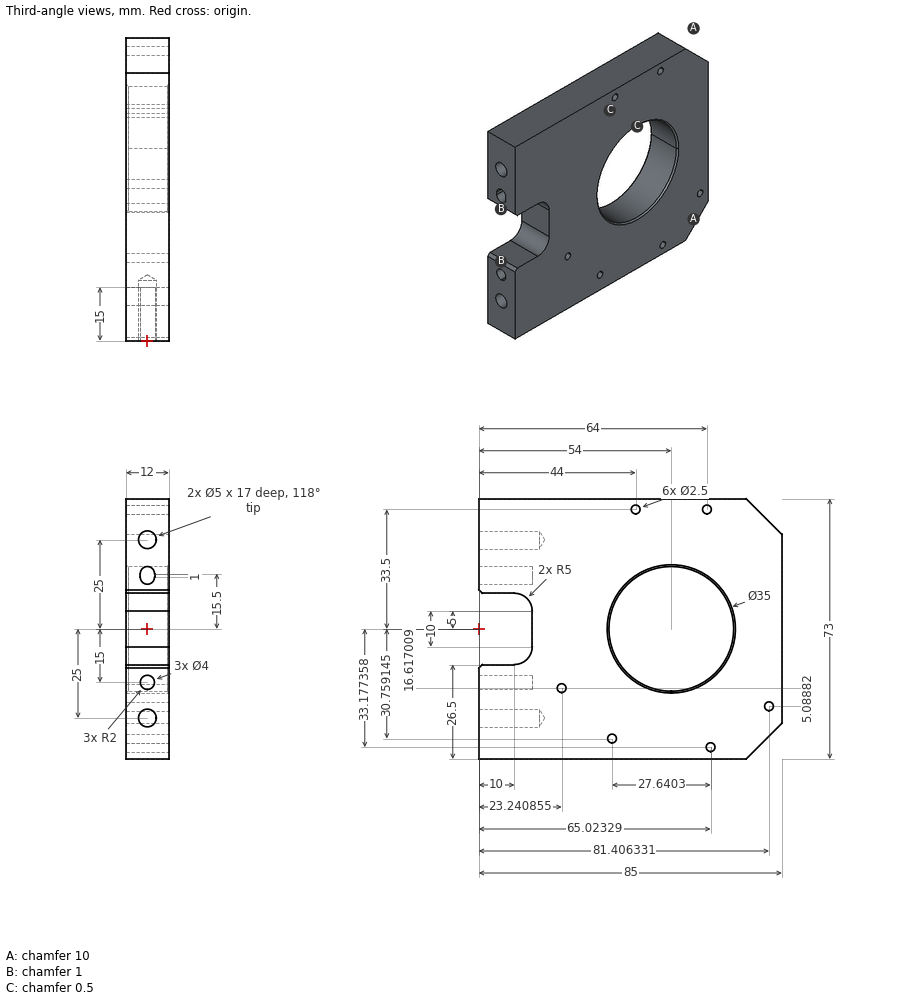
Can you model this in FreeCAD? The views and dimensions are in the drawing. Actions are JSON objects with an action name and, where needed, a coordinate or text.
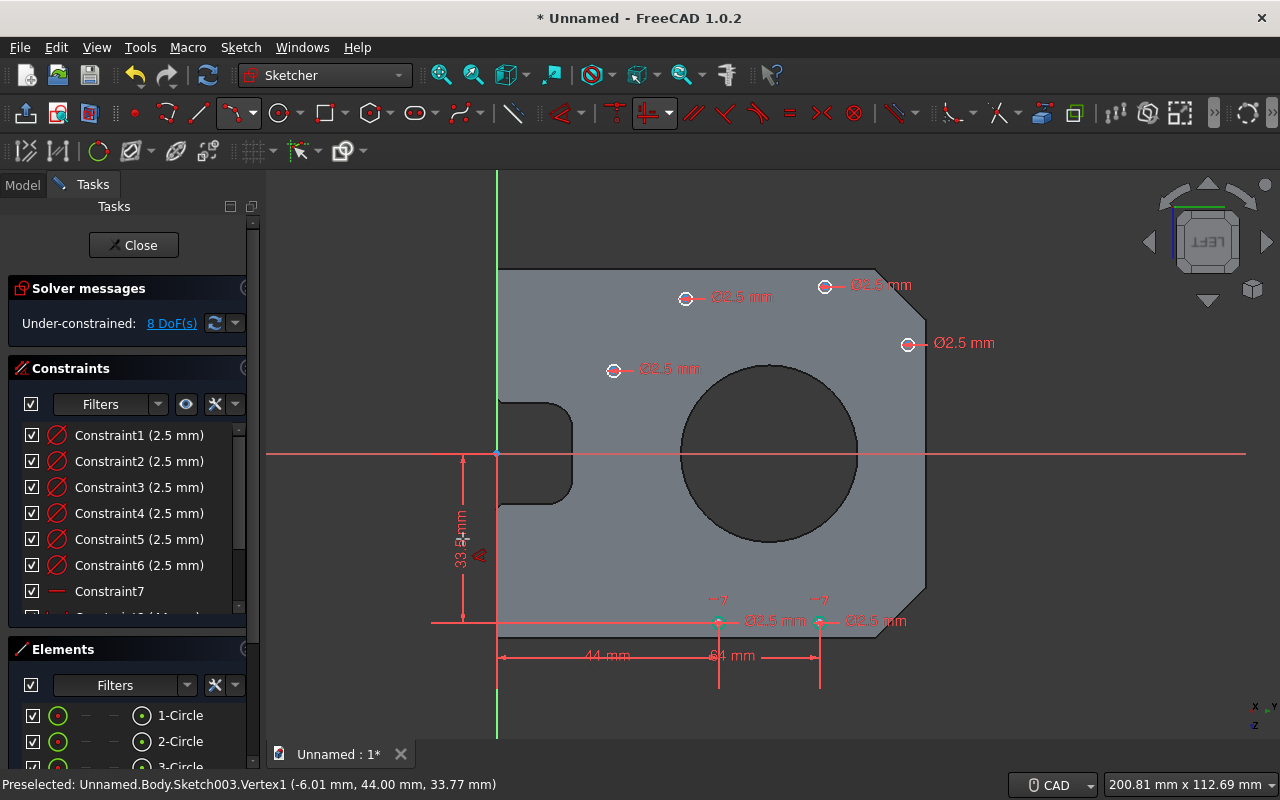
{"action": "left_click", "coordinate": [825, 287]}
{"action": "left_click", "coordinate": [661, 253]}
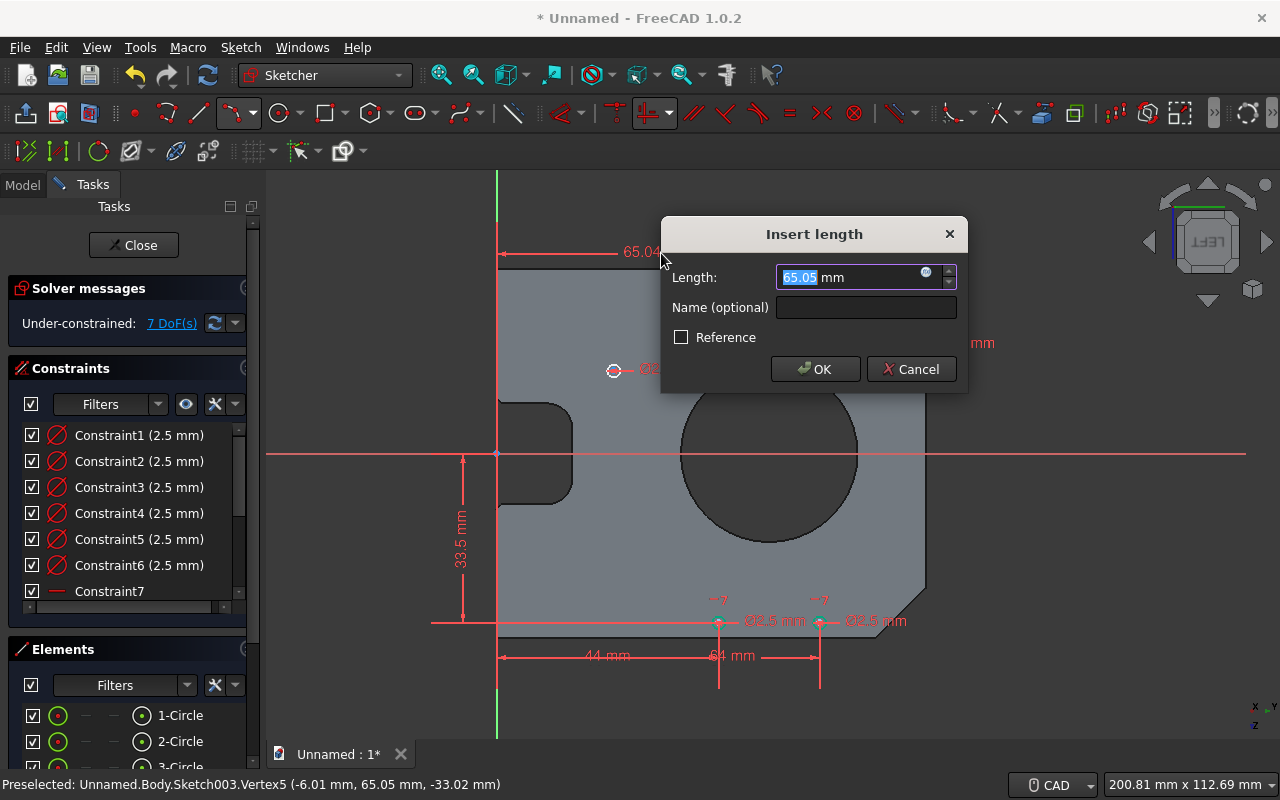
{"action": "type", "text": "65.02329"}
{"action": "key", "text": "Return"}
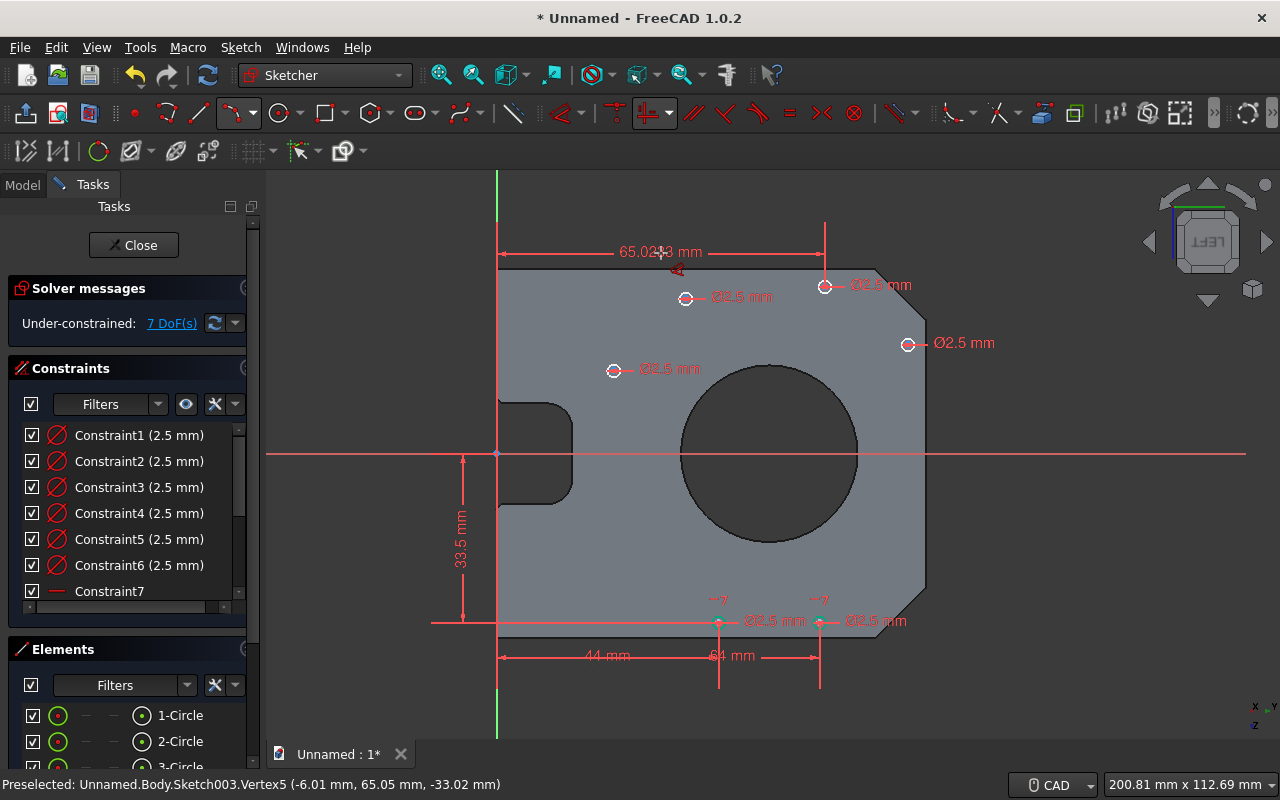
{"action": "left_click", "coordinate": [686, 299]}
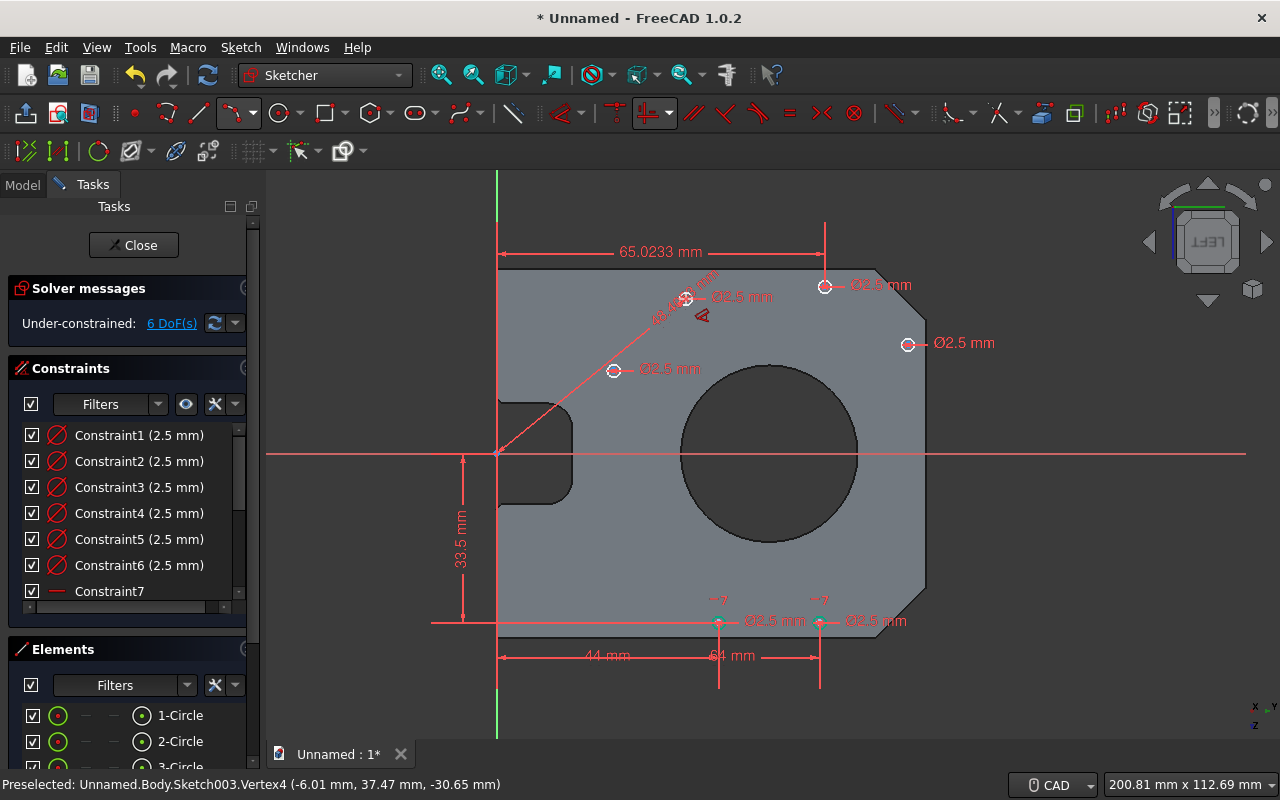
{"action": "left_click", "coordinate": [825, 287]}
{"action": "left_click", "coordinate": [755, 253]}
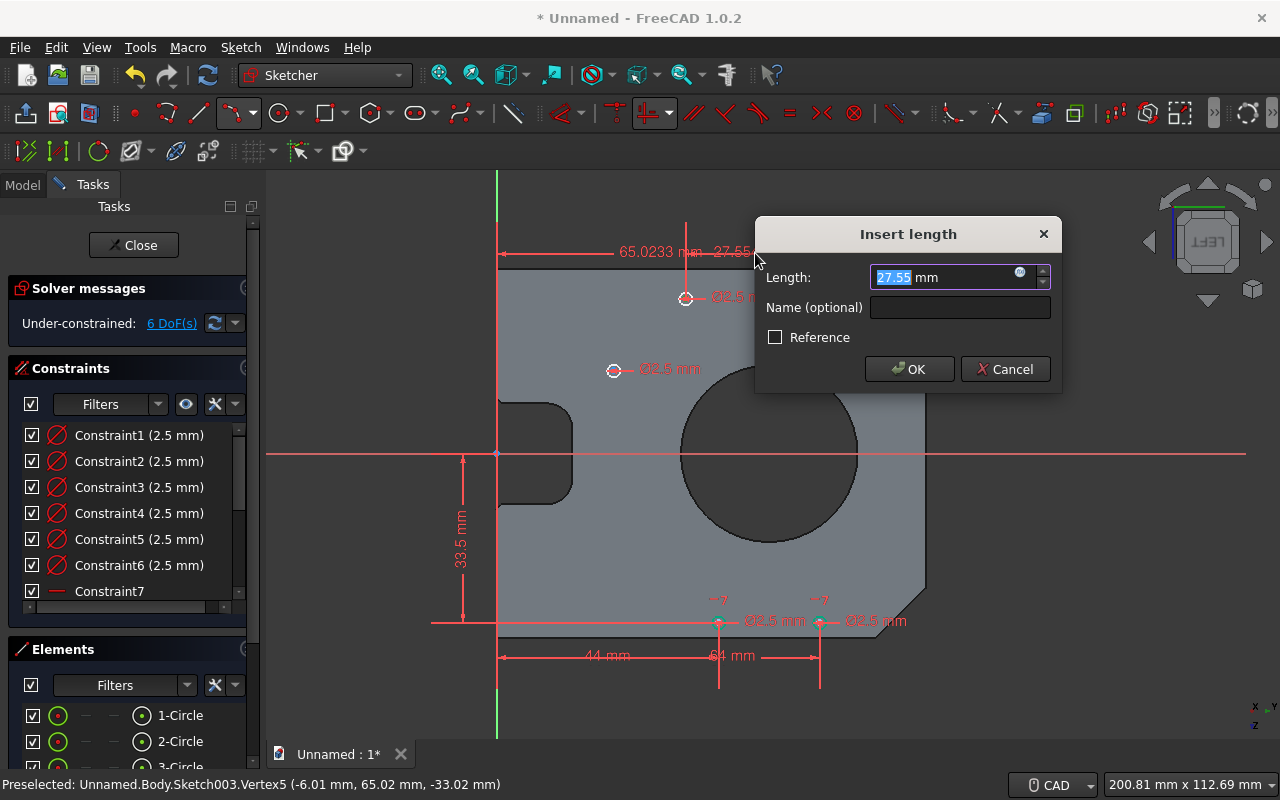
{"action": "type", "text": "27.6403"}
{"action": "key", "text": "Return"}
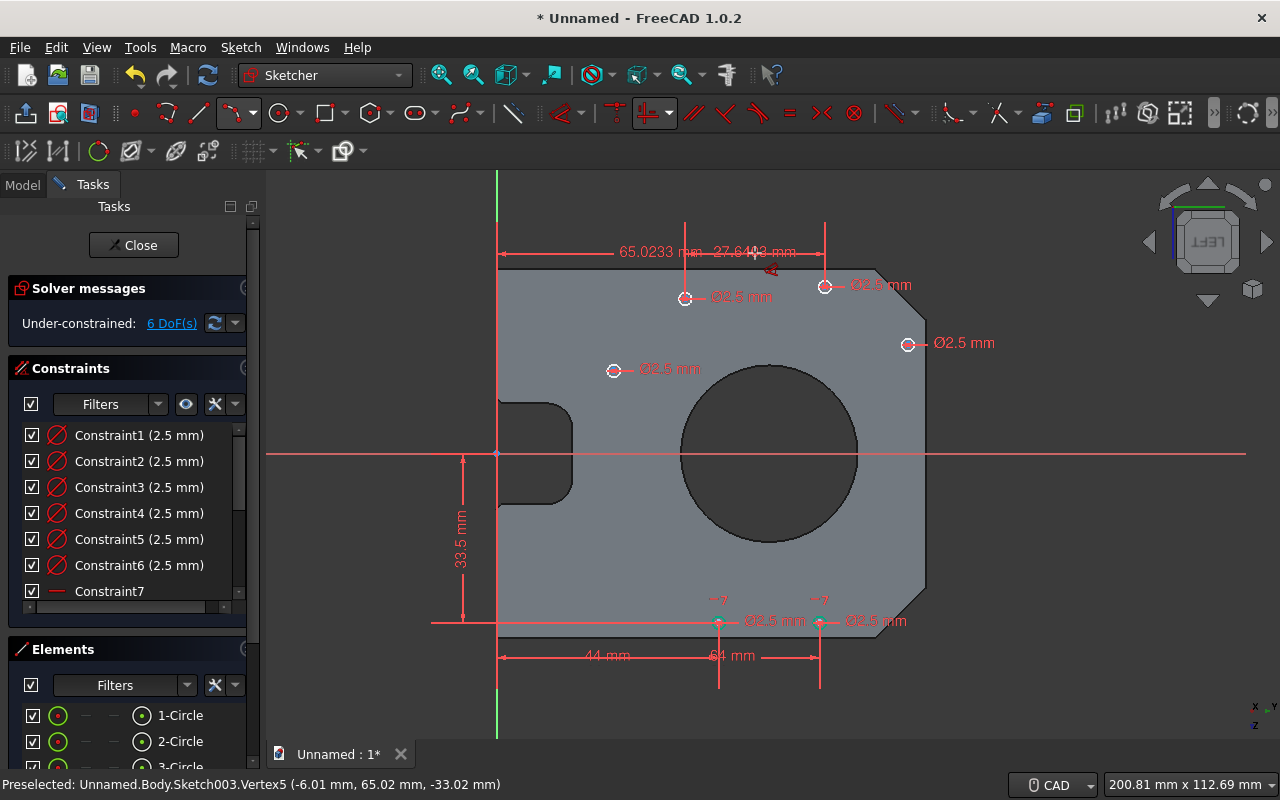
{"action": "scroll", "coordinate": [614, 371], "scroll_direction": "up", "scroll_amount": 3}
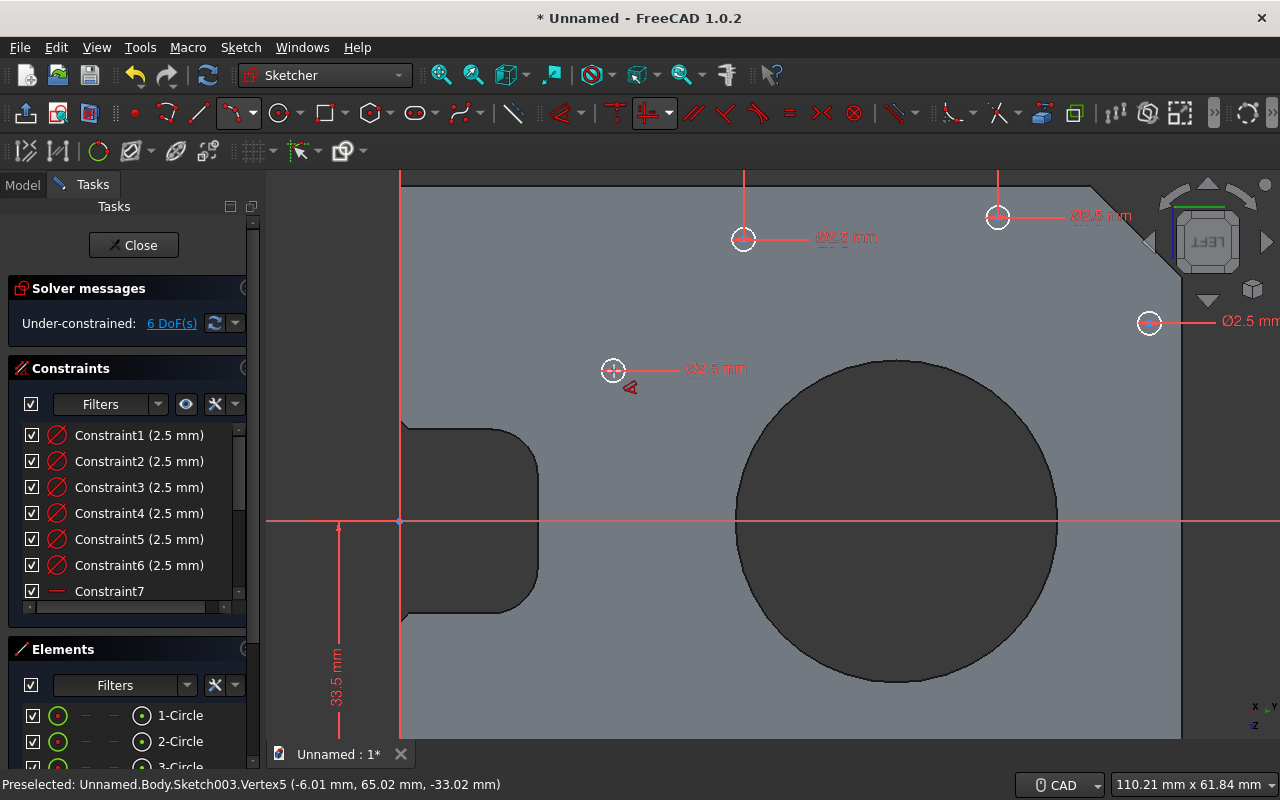
{"action": "left_click", "coordinate": [613, 371]}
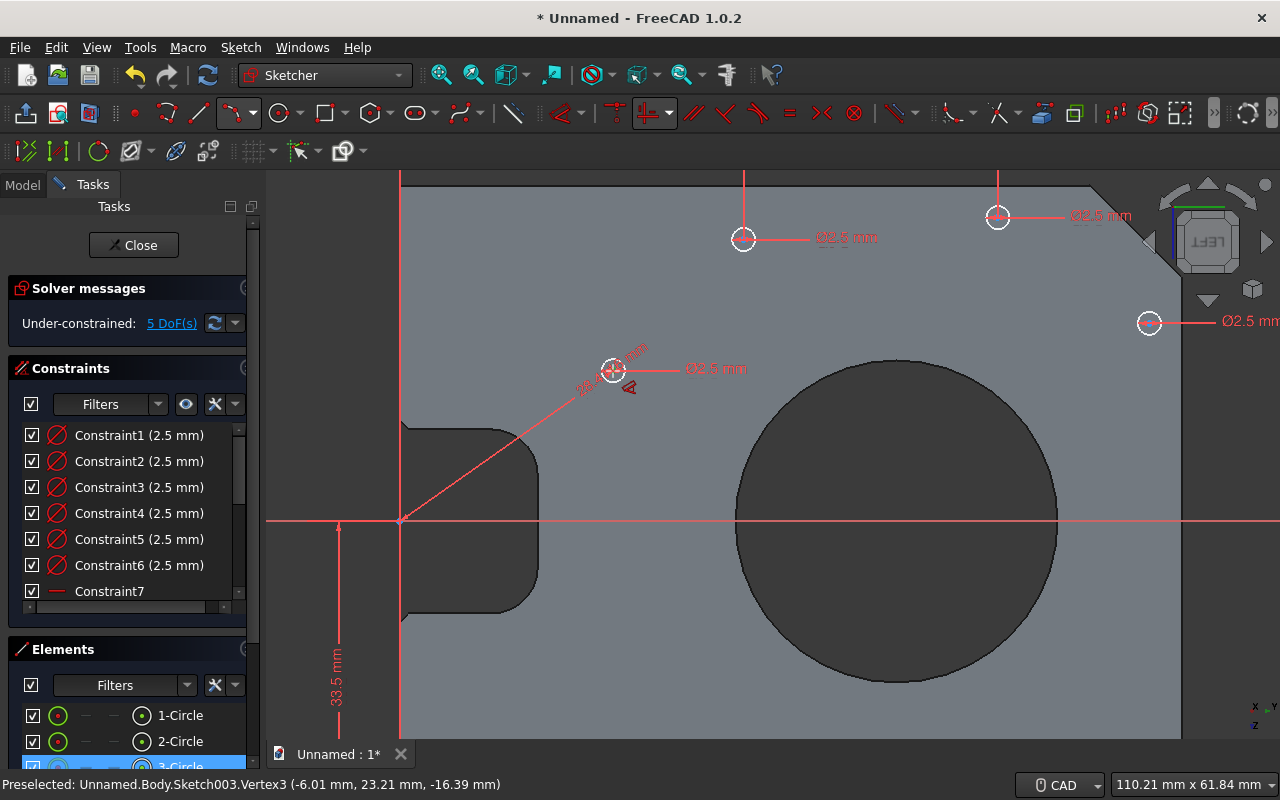
{"action": "scroll", "coordinate": [613, 371], "scroll_direction": "down", "scroll_amount": 3}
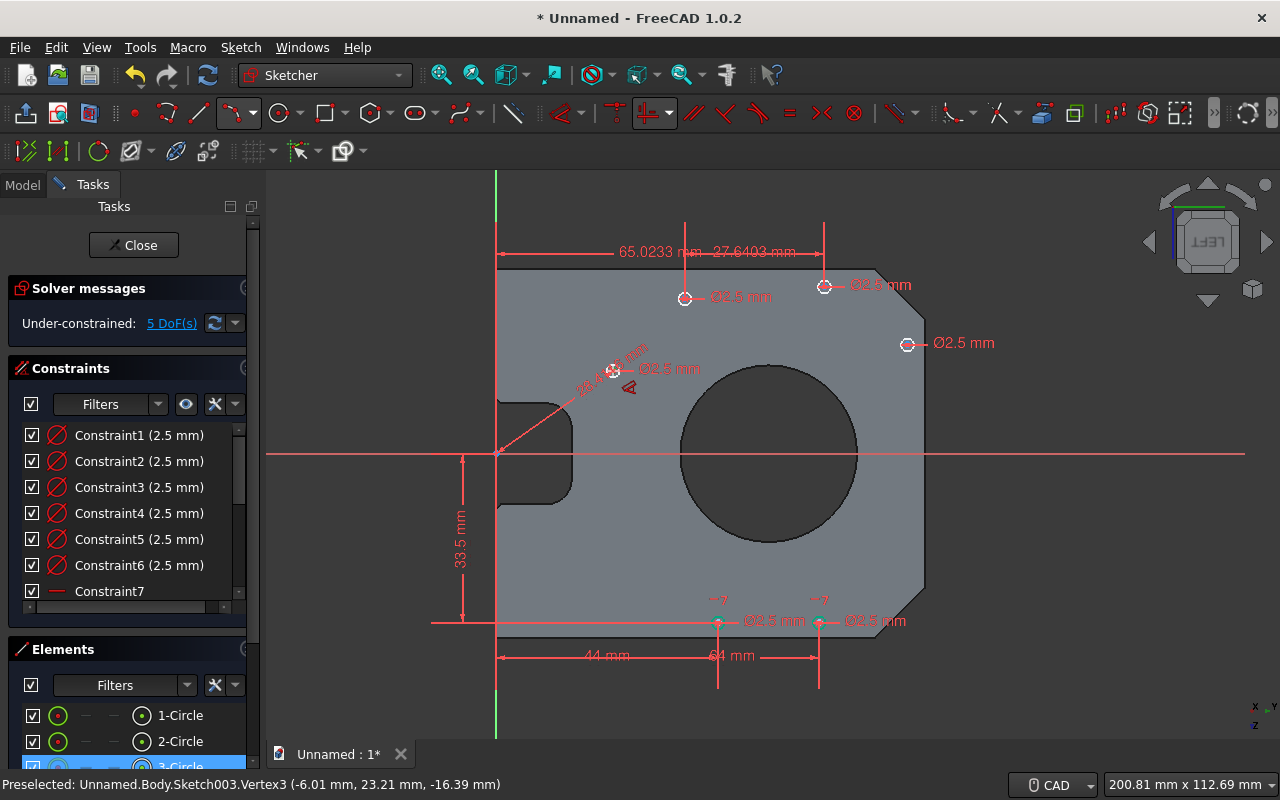
{"action": "scroll", "coordinate": [908, 345], "scroll_direction": "up", "scroll_amount": 3}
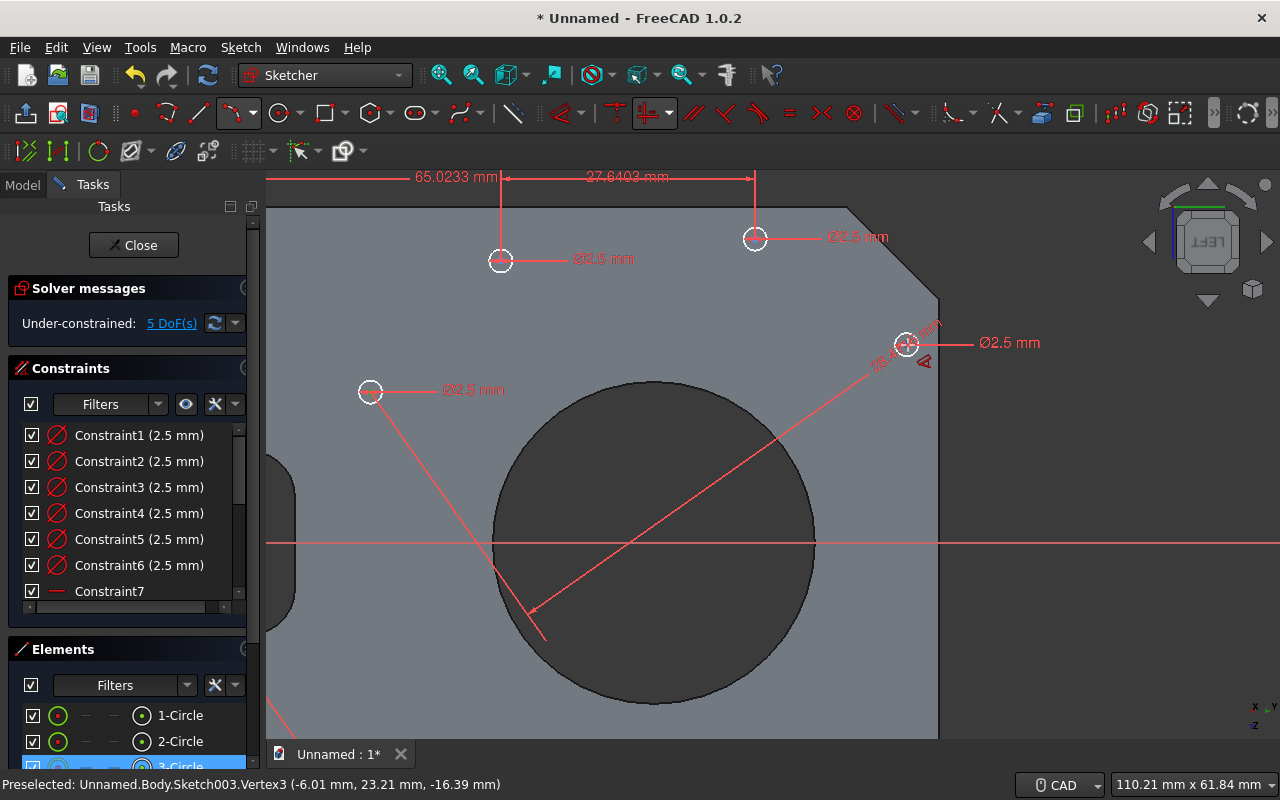
{"action": "left_click", "coordinate": [907, 345]}
{"action": "left_click", "coordinate": [941, 368]}